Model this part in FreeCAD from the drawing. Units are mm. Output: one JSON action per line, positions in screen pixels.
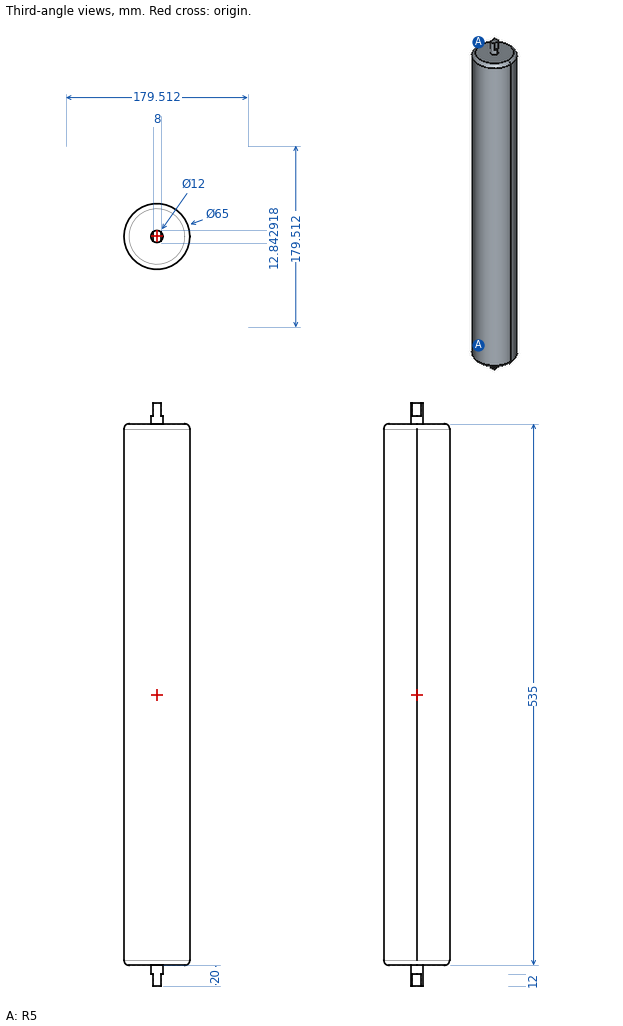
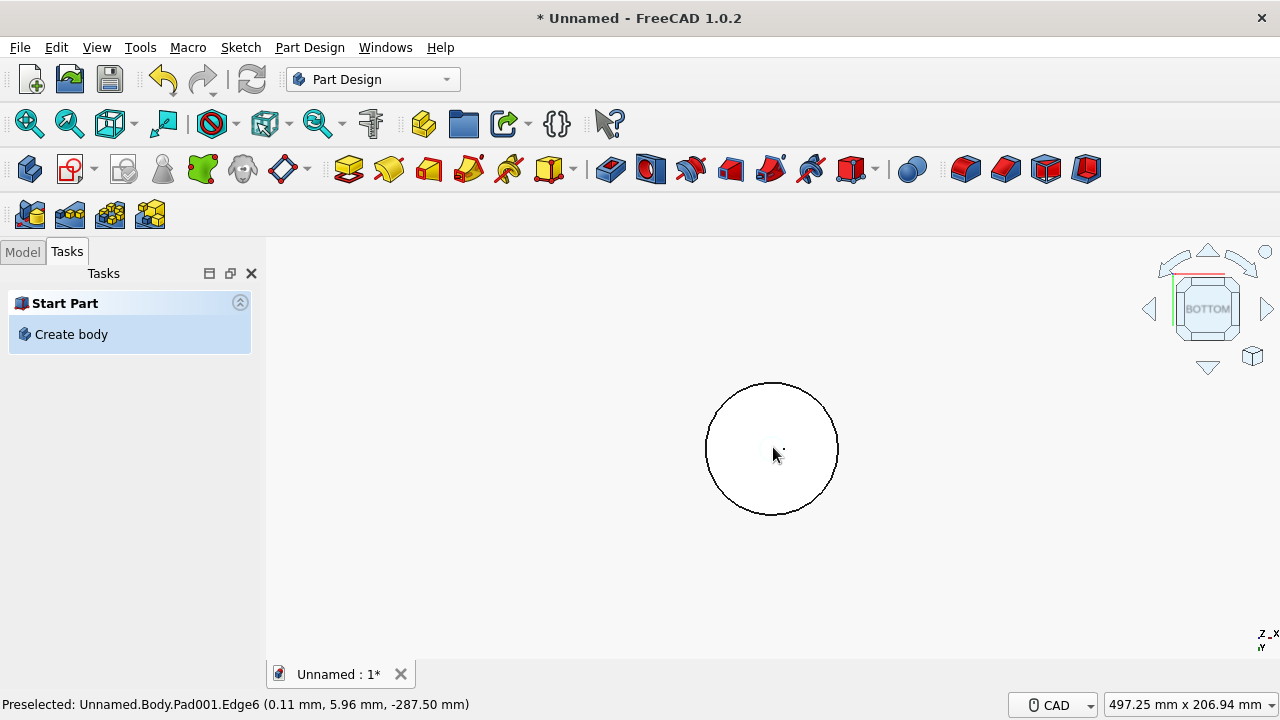
{"action": "left_click", "coordinate": [772, 448]}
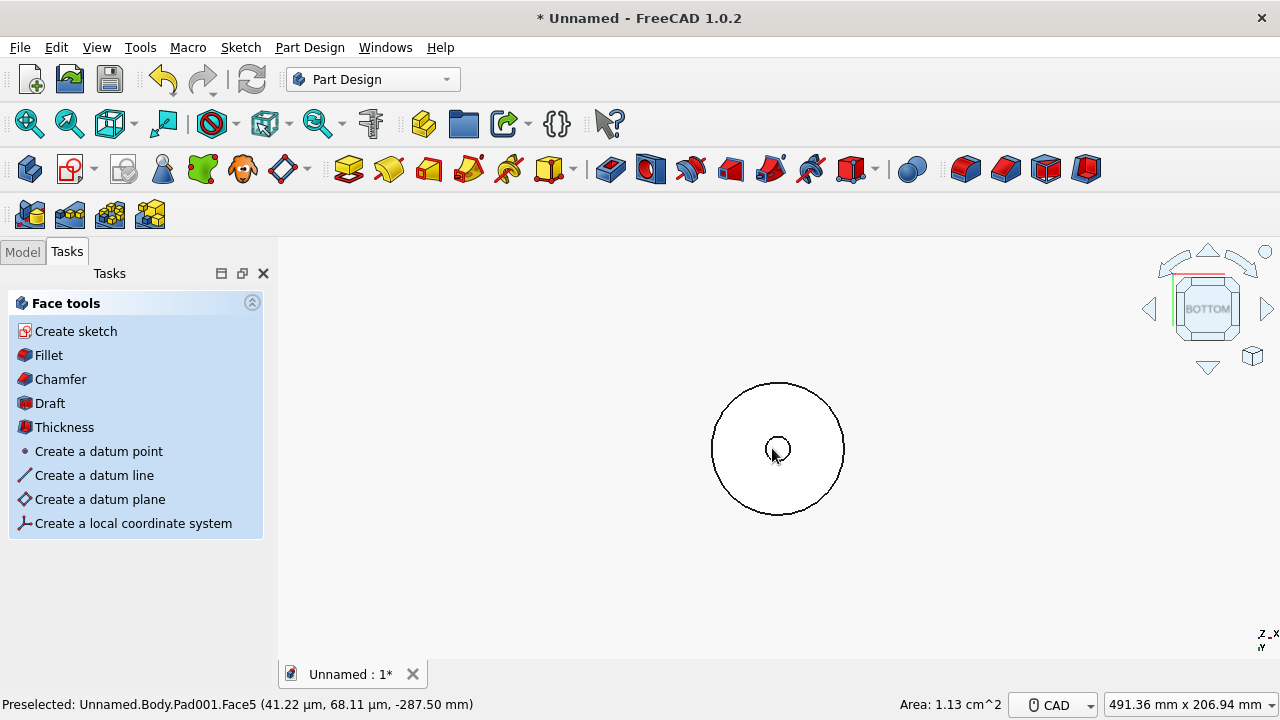
{"action": "left_click", "coordinate": [70, 170]}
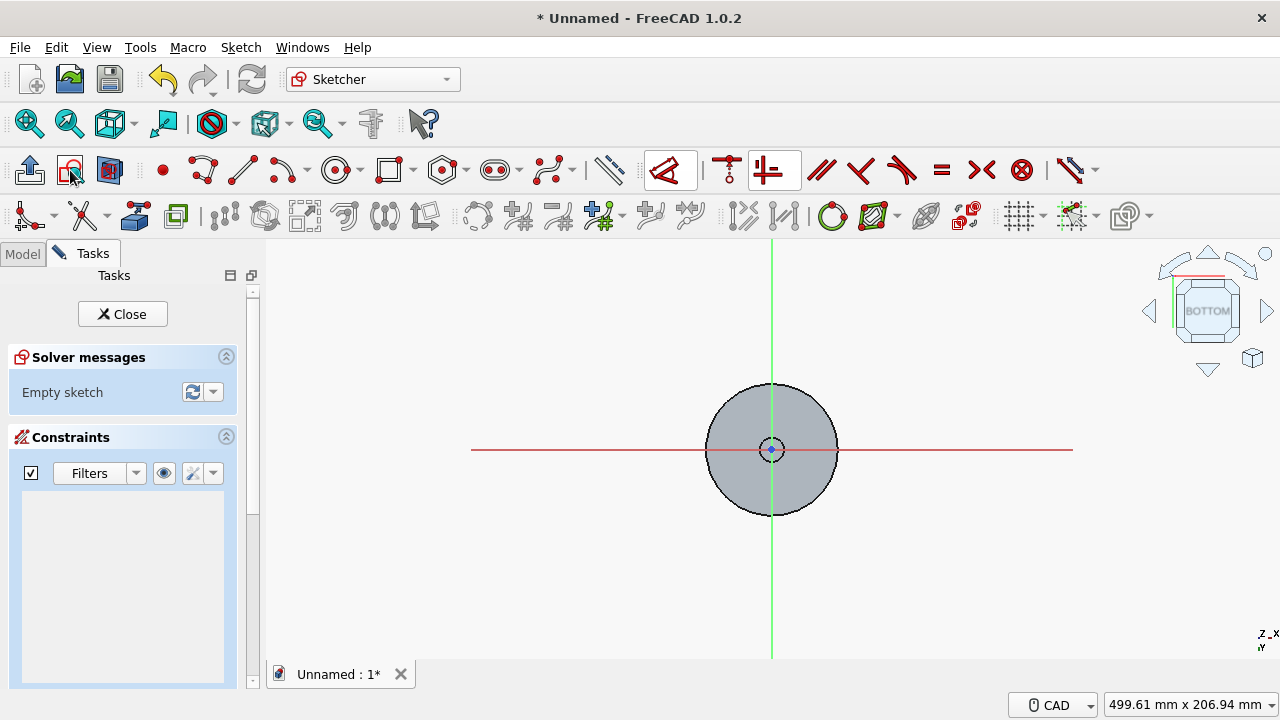
{"action": "scroll", "coordinate": [567, 447], "scroll_direction": "down", "scroll_amount": 2}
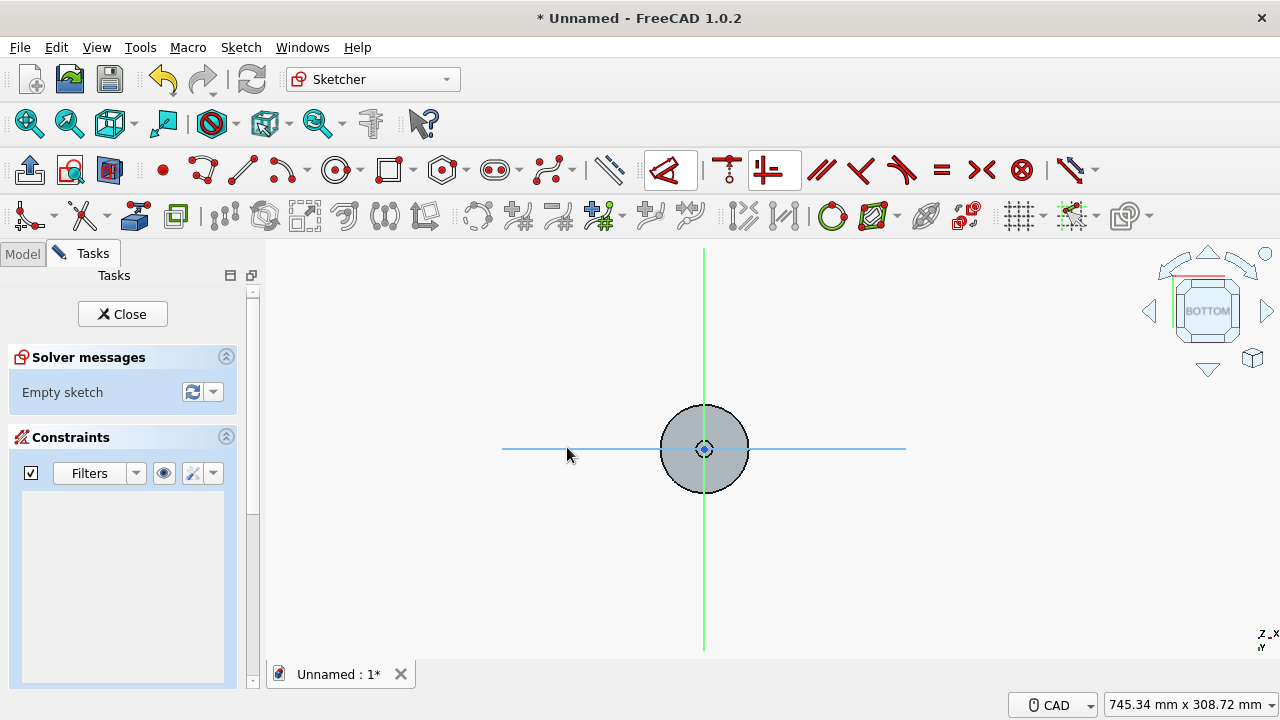
{"action": "key", "text": "g v"}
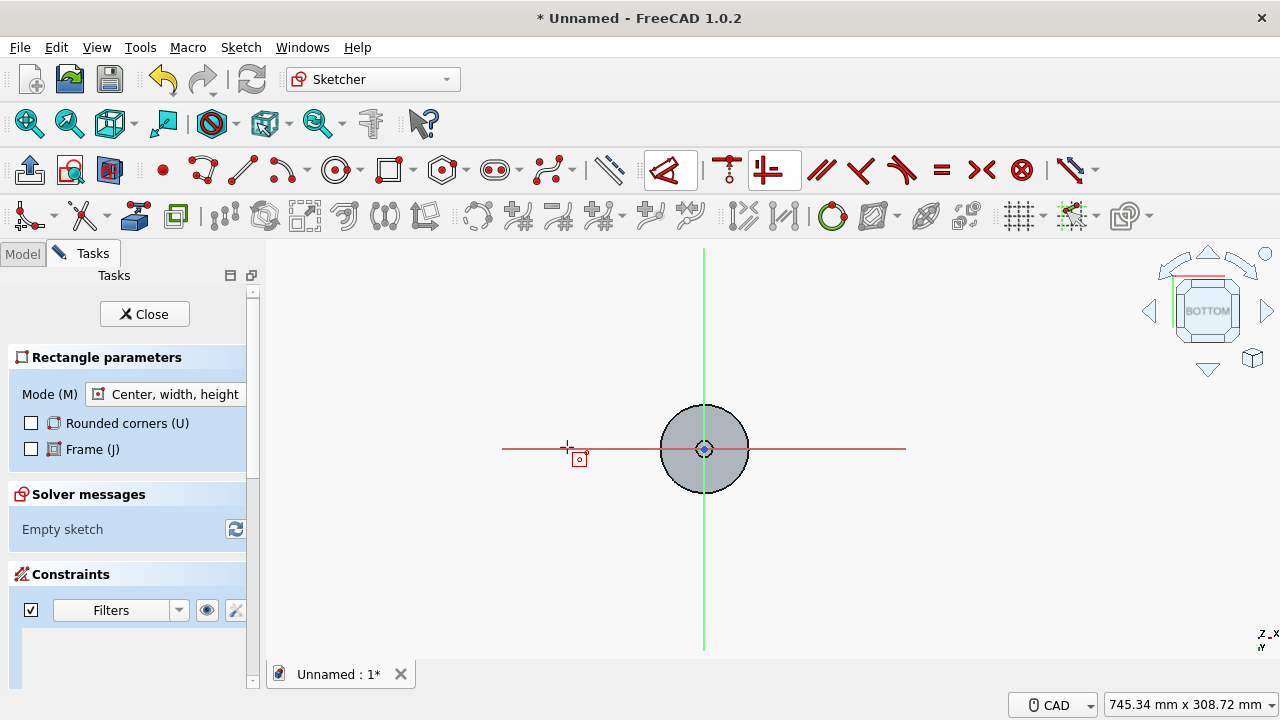
{"action": "left_click", "coordinate": [704, 449]}
{"action": "left_click", "coordinate": [827, 327]}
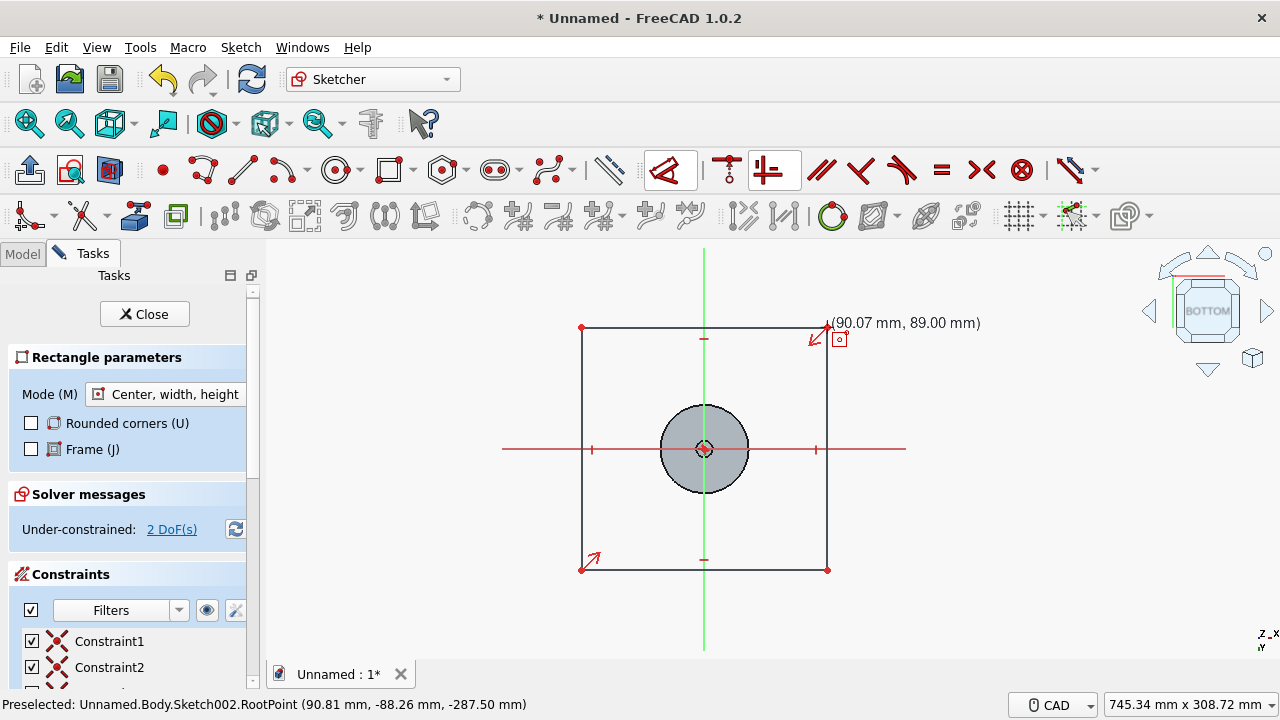
{"action": "scroll", "coordinate": [704, 449], "scroll_direction": "up", "scroll_amount": 6}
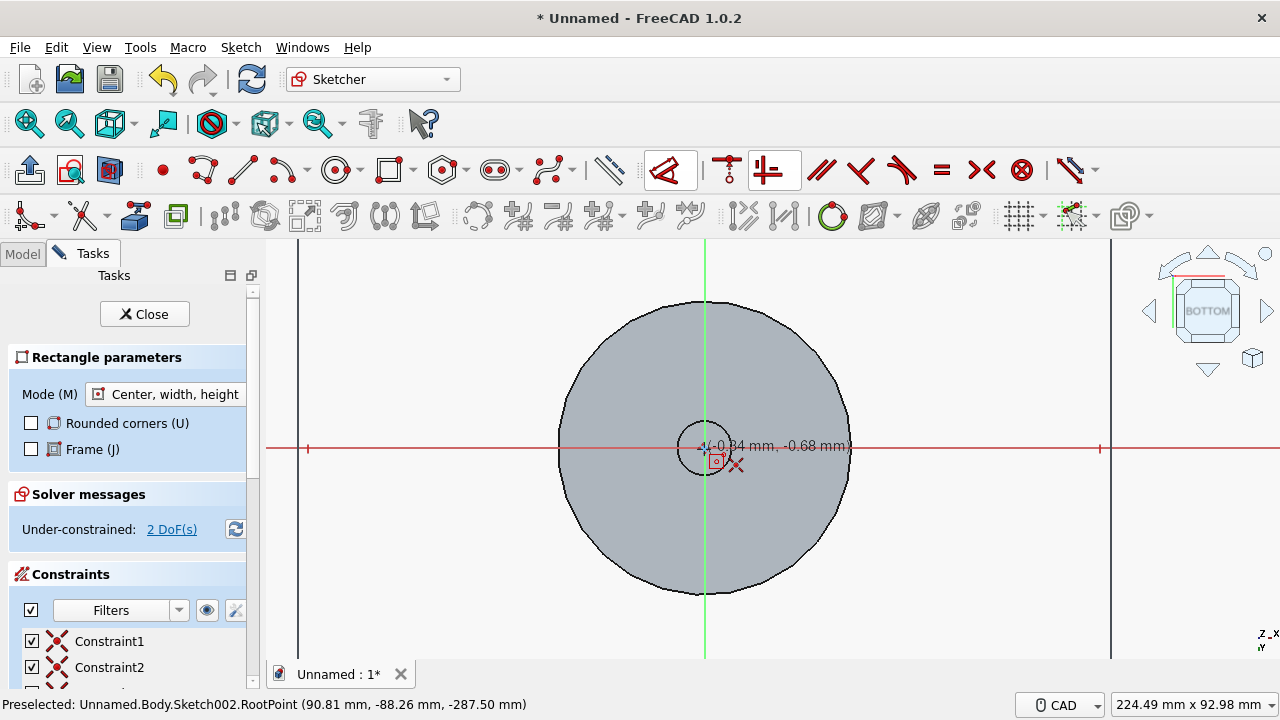
{"action": "left_click", "coordinate": [705, 448]}
{"action": "left_click", "coordinate": [723, 419]}
{"action": "key", "text": "Escape"}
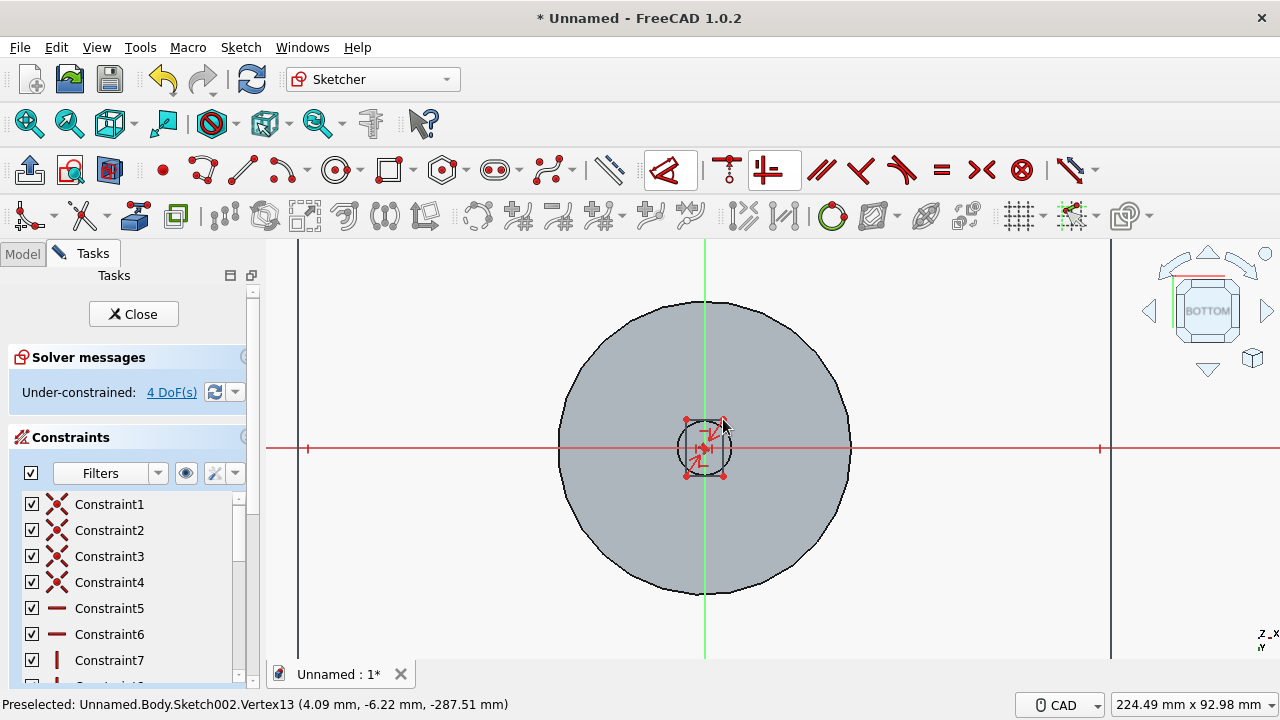
{"action": "left_click", "coordinate": [701, 476]}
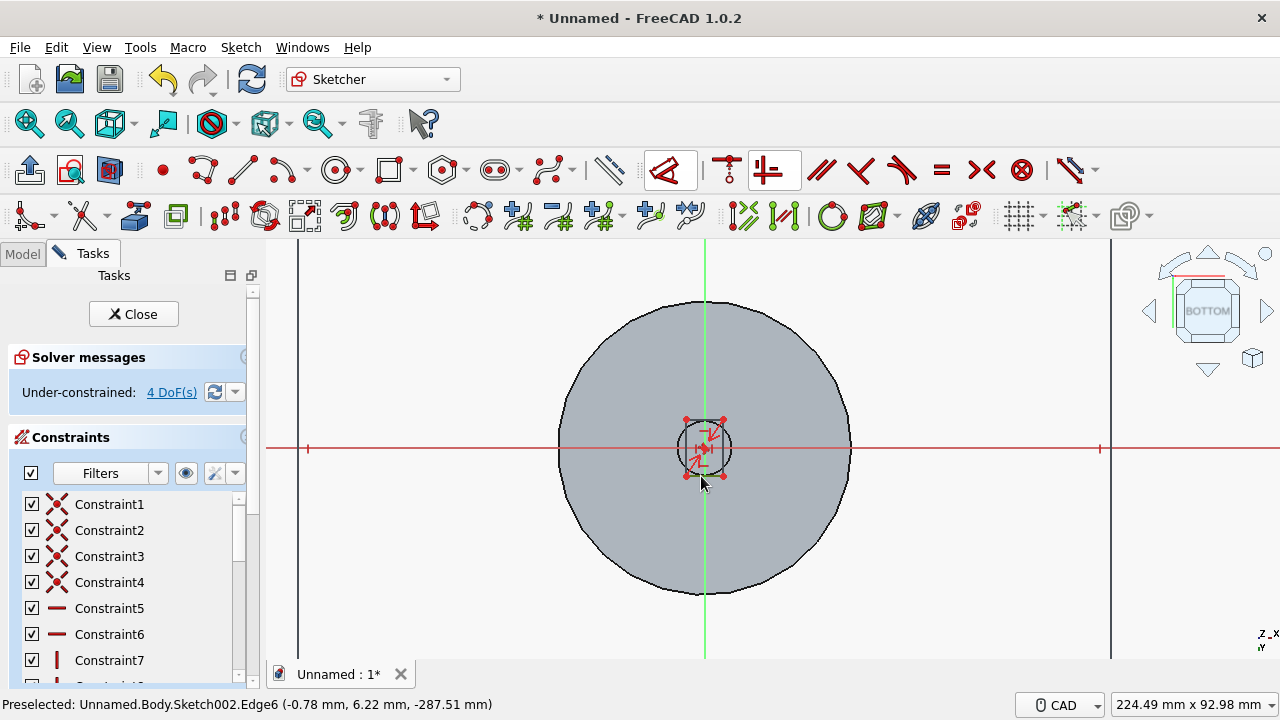
{"action": "key", "text": "l"}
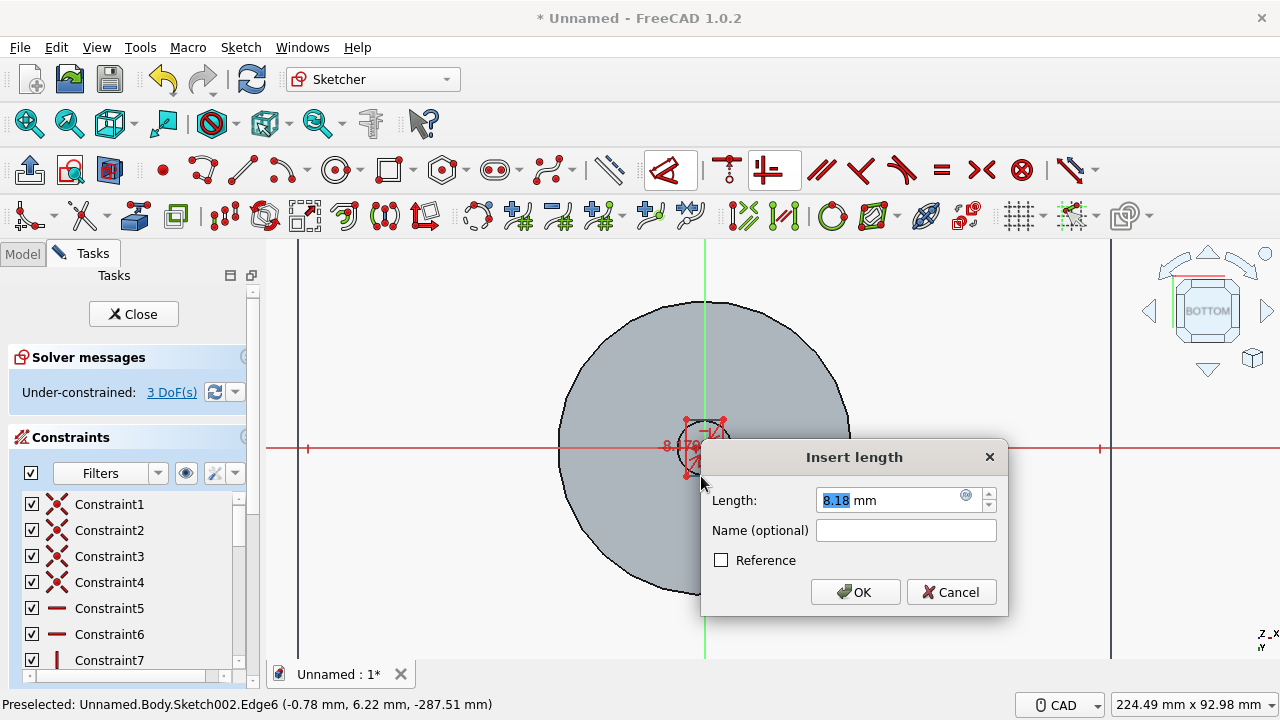
{"action": "type", "text": "8"}
{"action": "key", "text": "Return"}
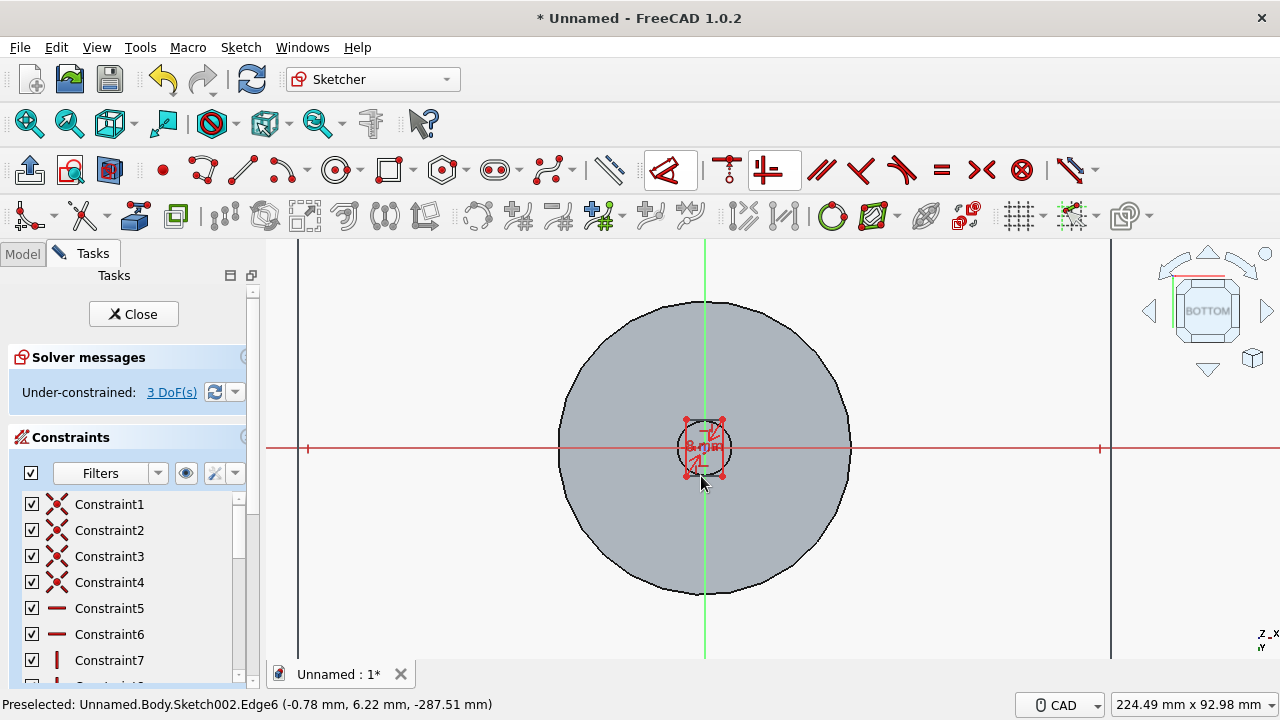
{"action": "scroll", "coordinate": [704, 449], "scroll_direction": "down", "scroll_amount": 6}